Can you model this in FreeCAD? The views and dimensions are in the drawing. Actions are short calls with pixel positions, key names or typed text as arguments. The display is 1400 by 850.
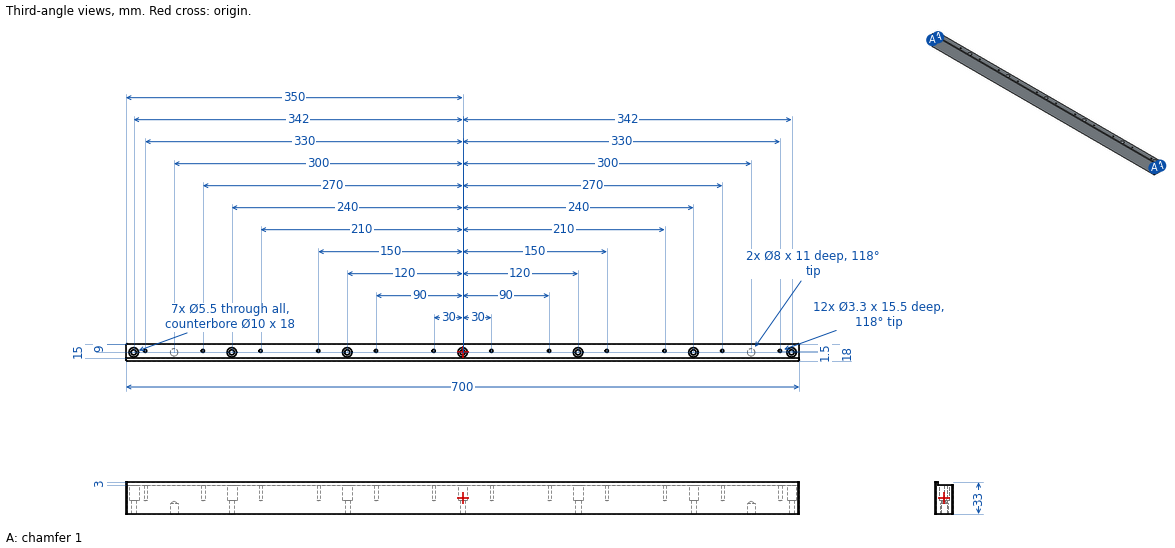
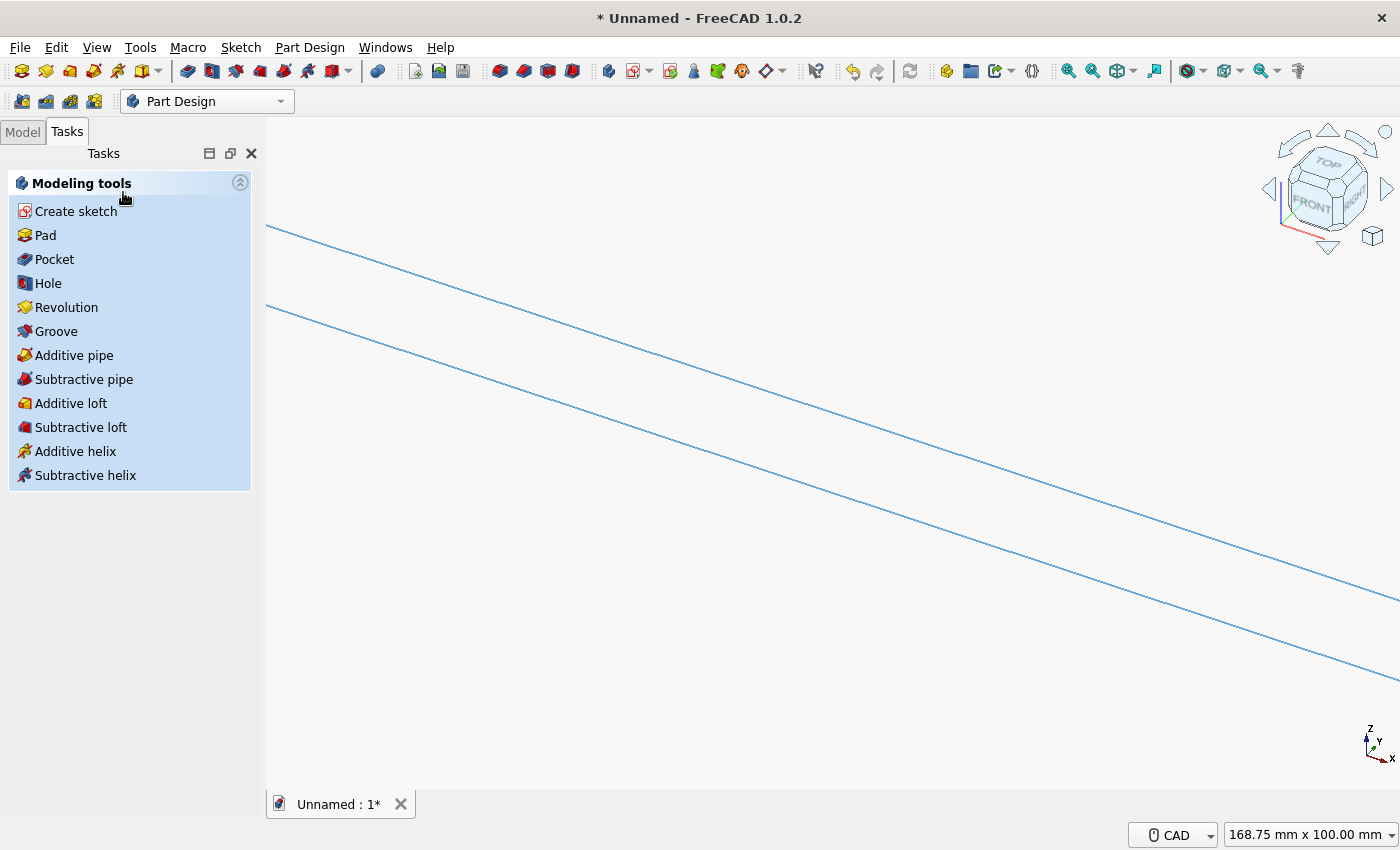
click(22, 72)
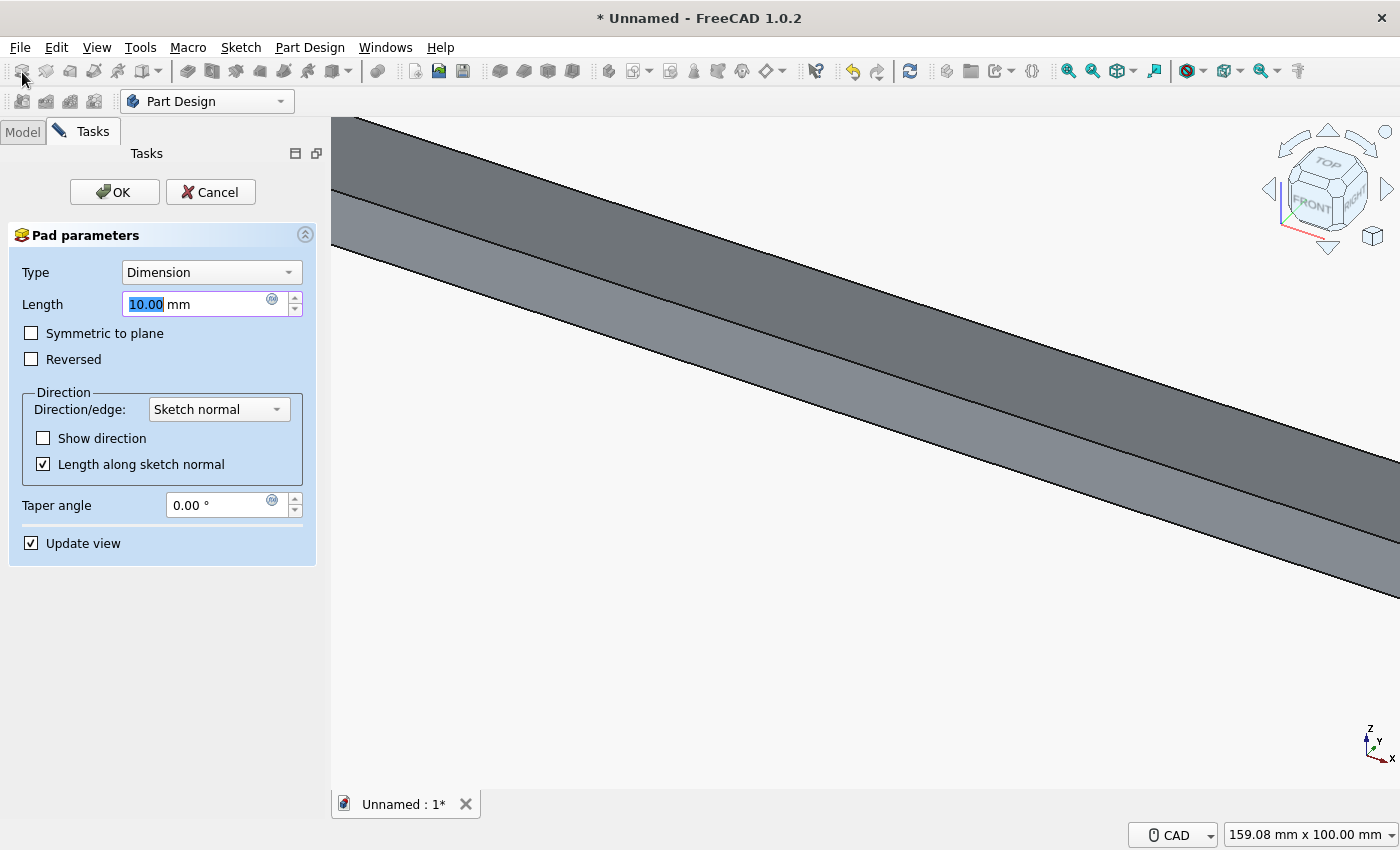
text(33)
key(Tab)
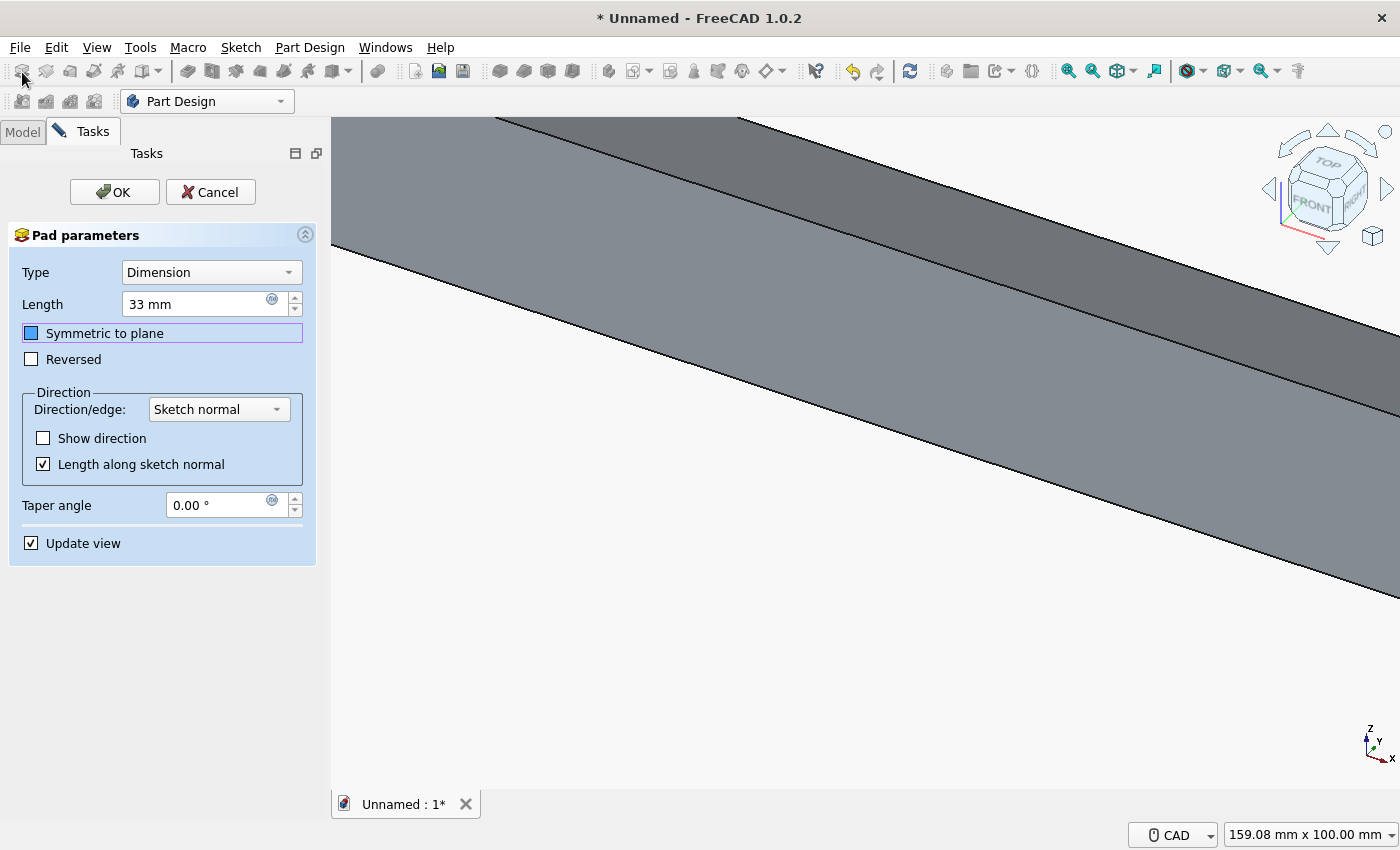
click(30, 333)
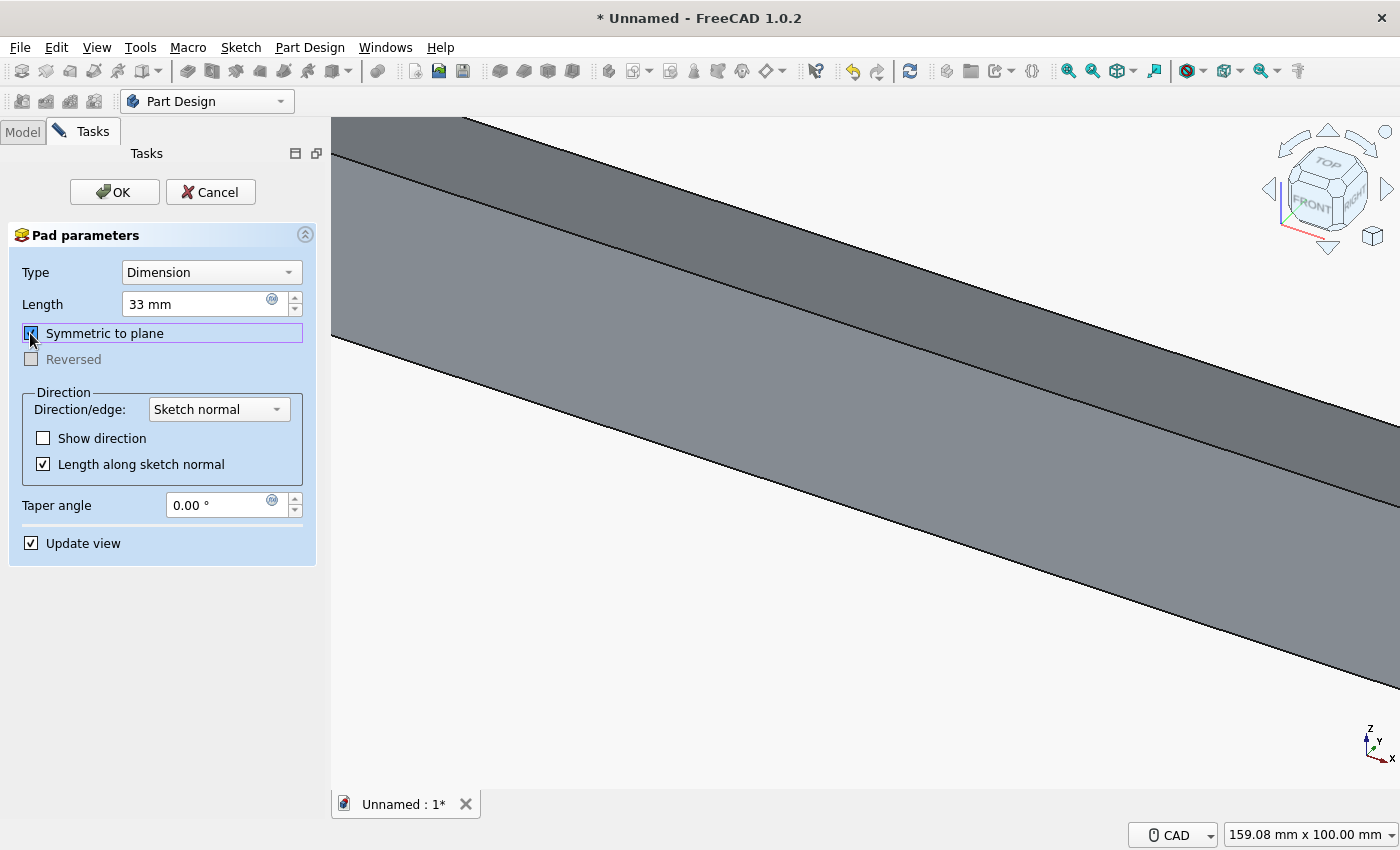
click(115, 192)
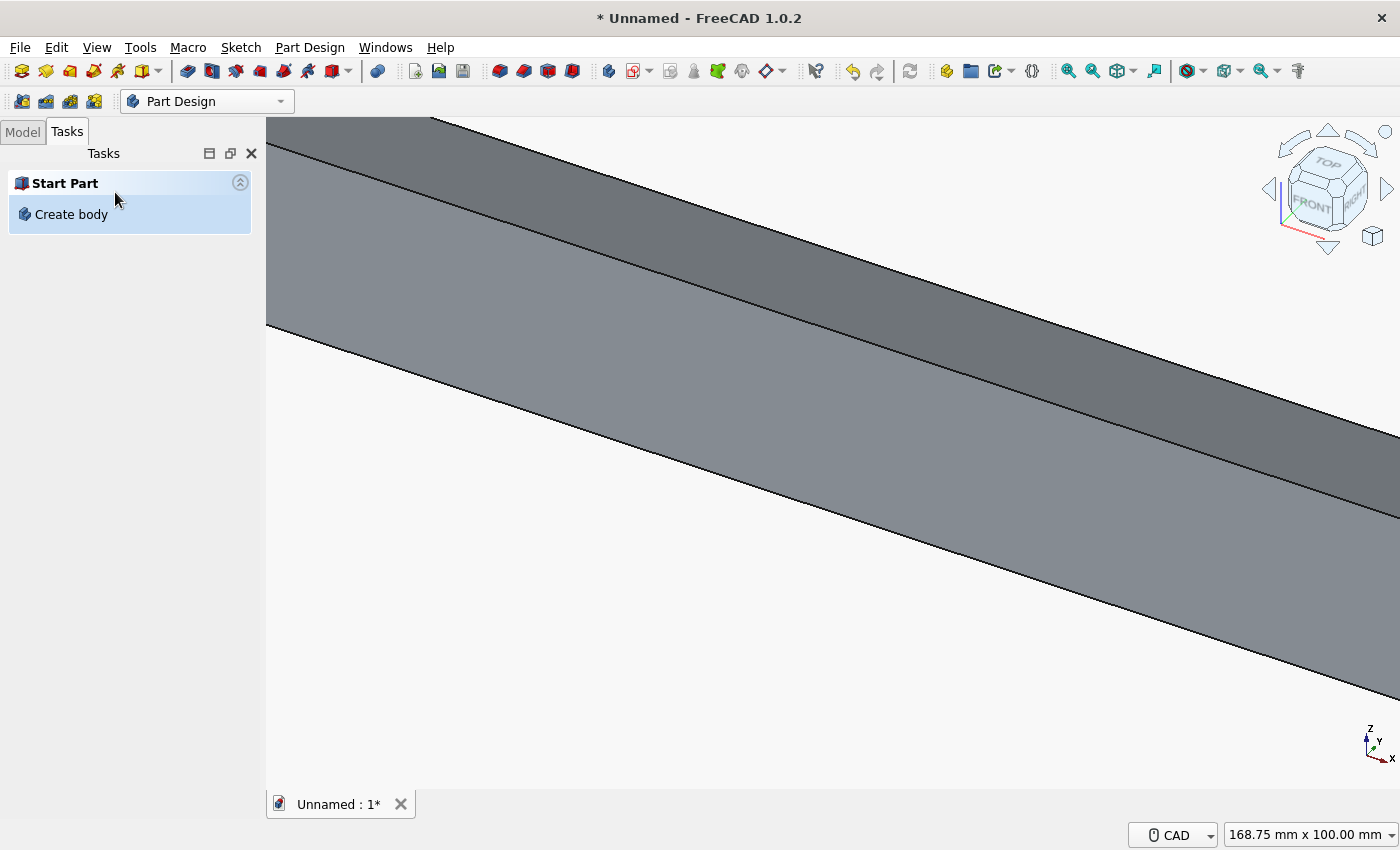
key(v)
key(f)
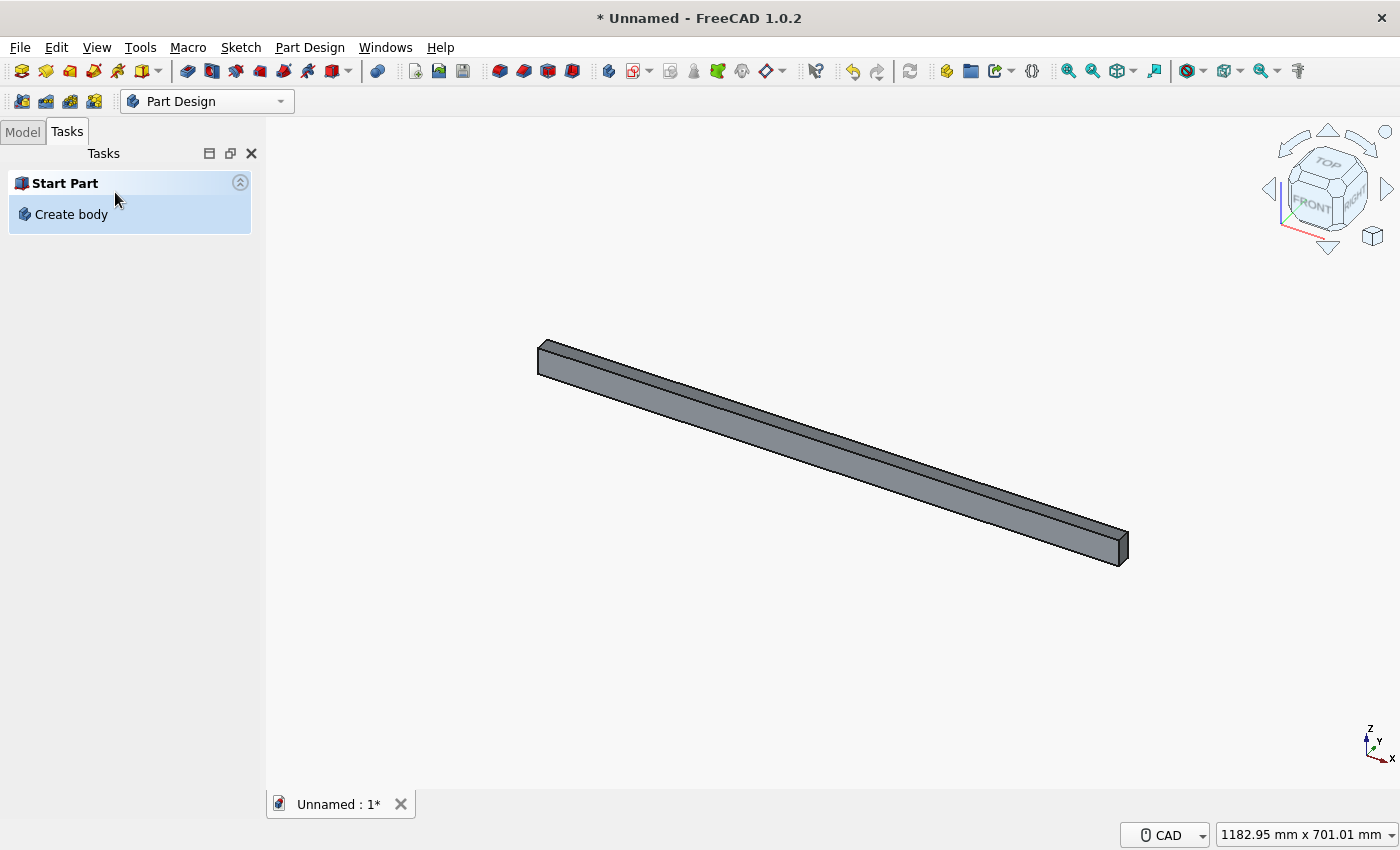
key(0)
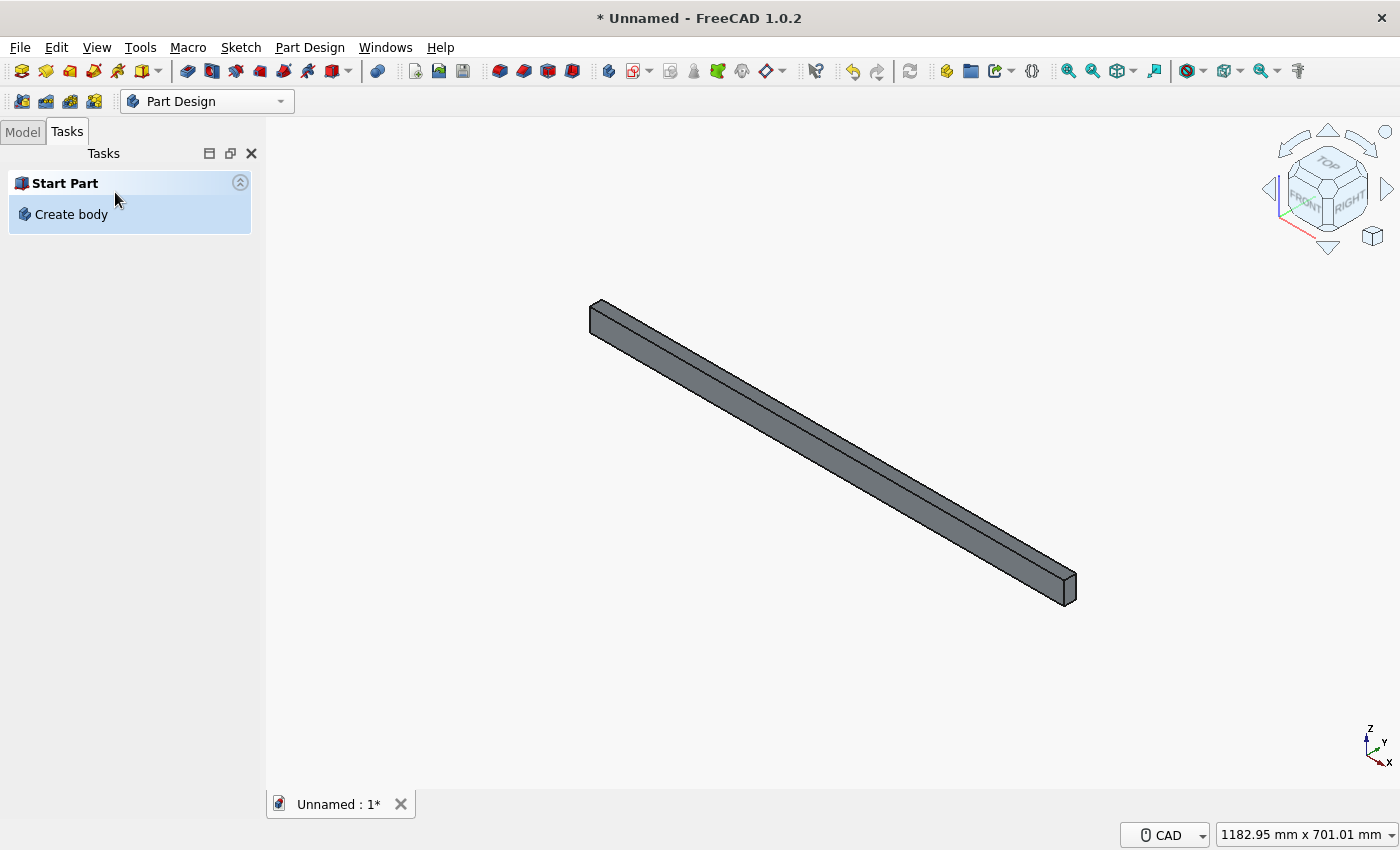
key(2)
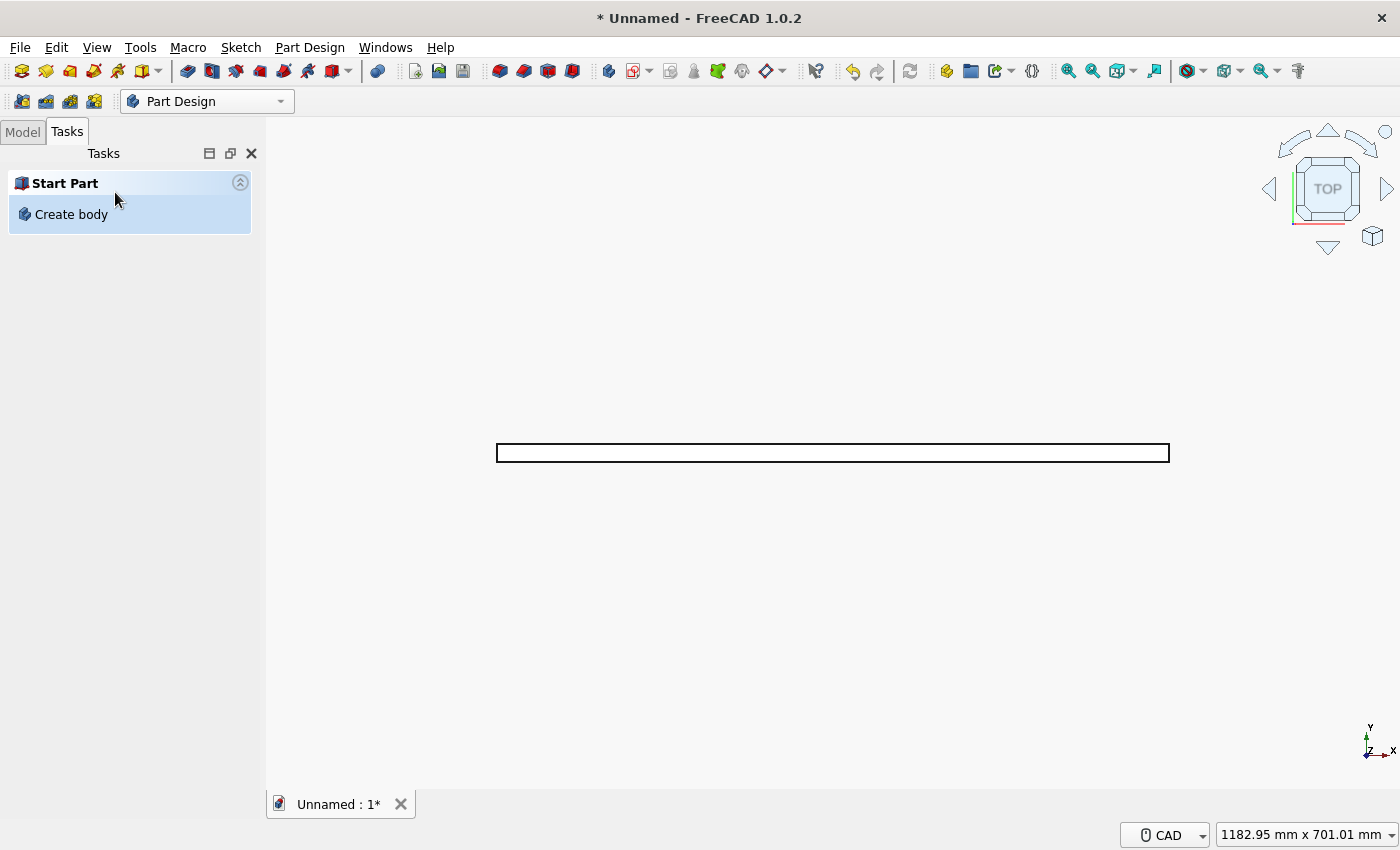
click(1121, 452)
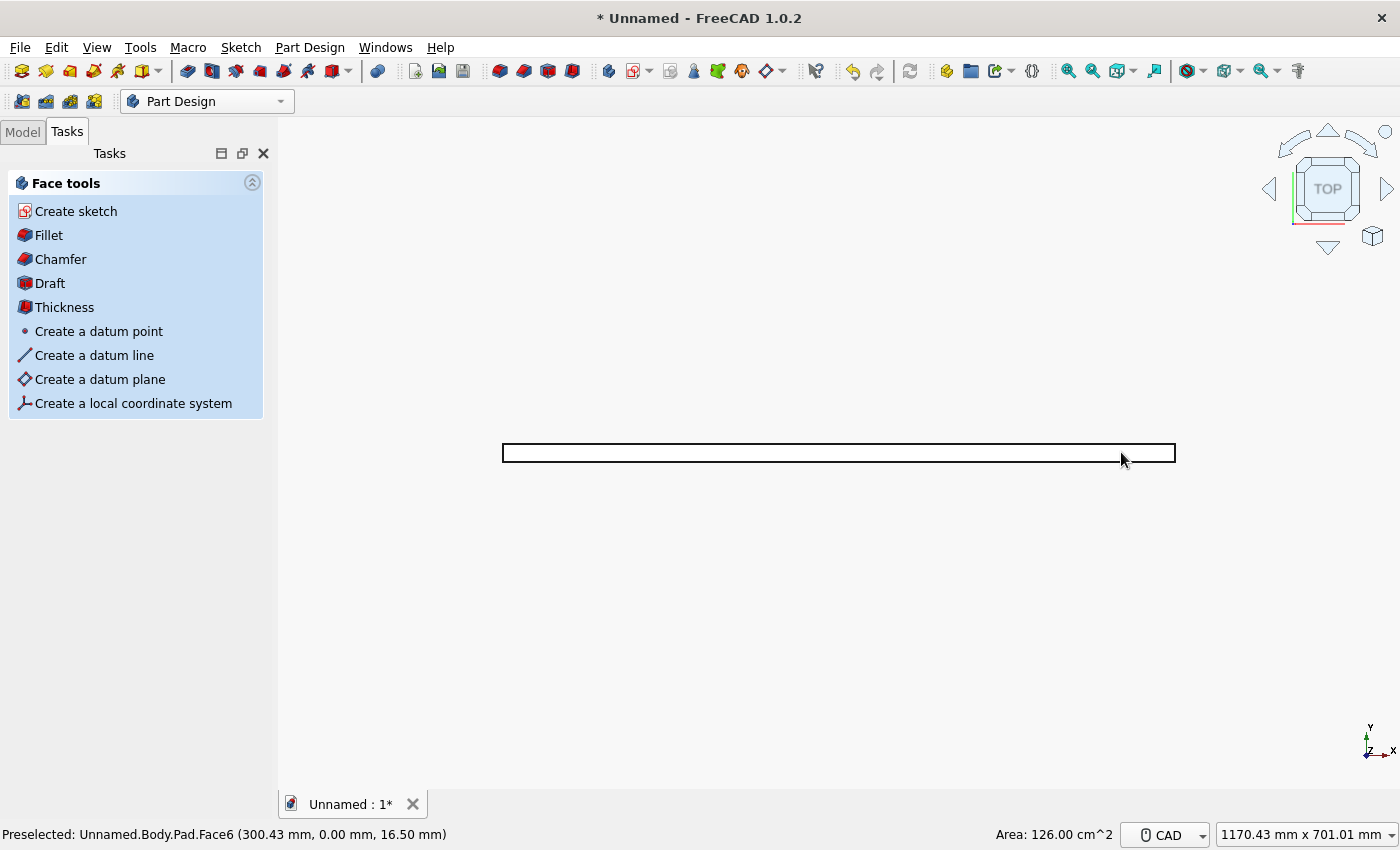
click(634, 72)